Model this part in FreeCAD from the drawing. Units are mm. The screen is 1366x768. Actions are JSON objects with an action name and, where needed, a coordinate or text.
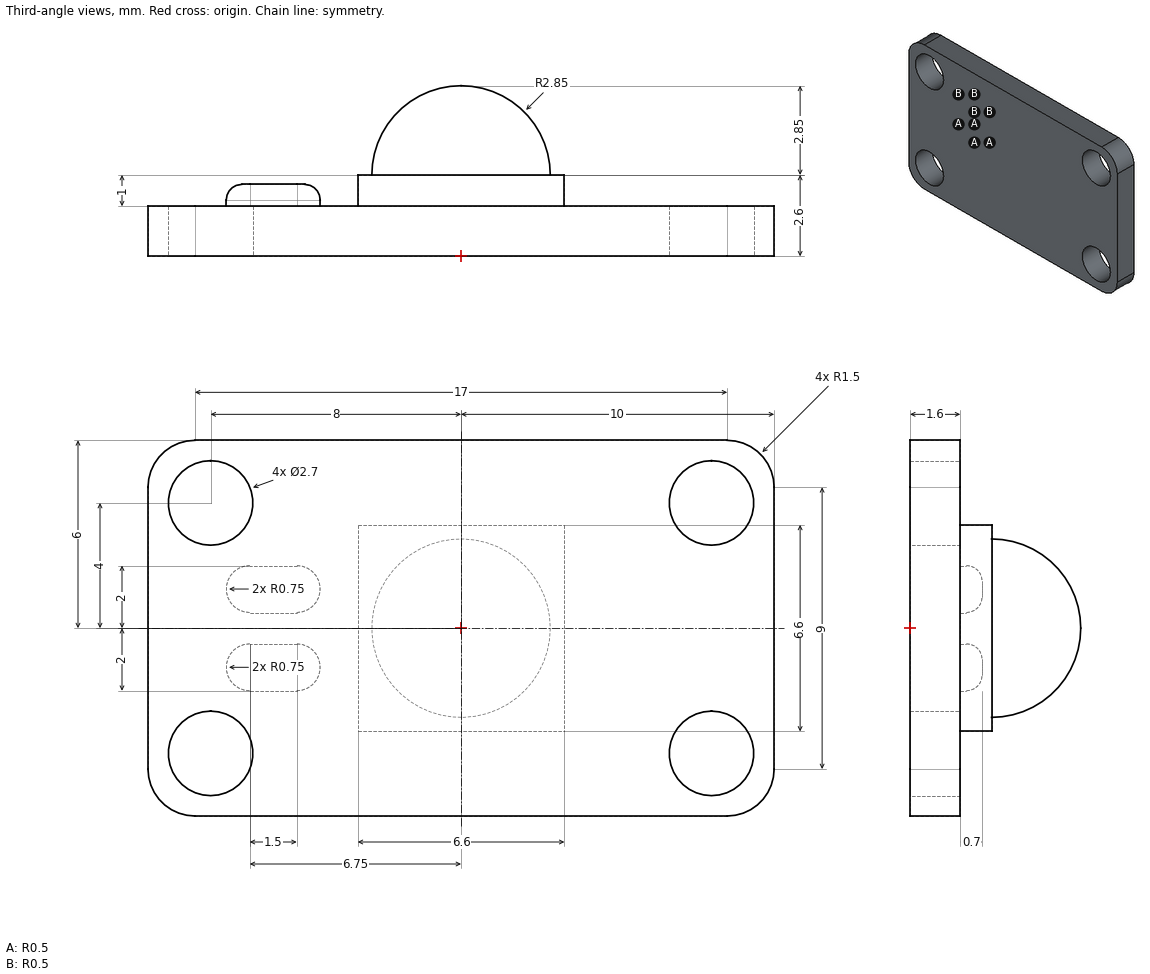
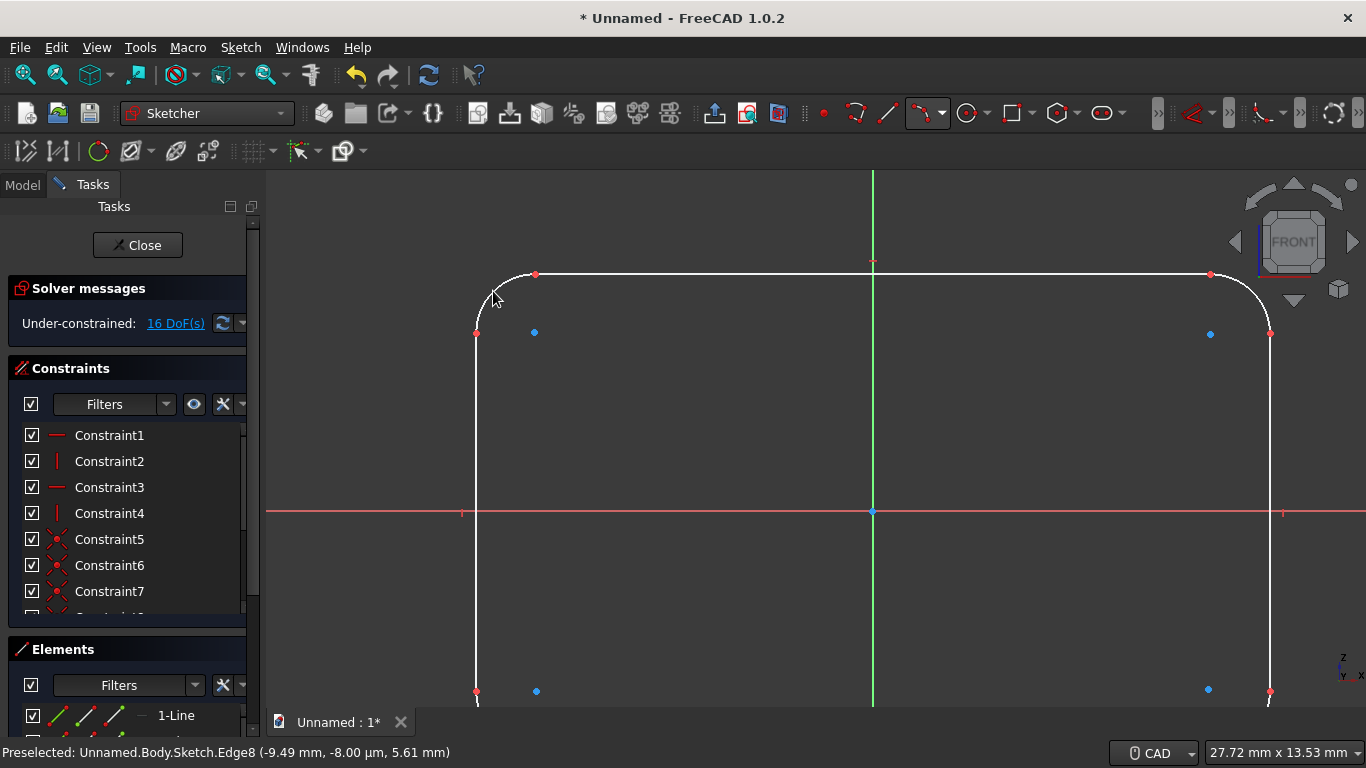
{"action": "left_click", "coordinate": [738, 274]}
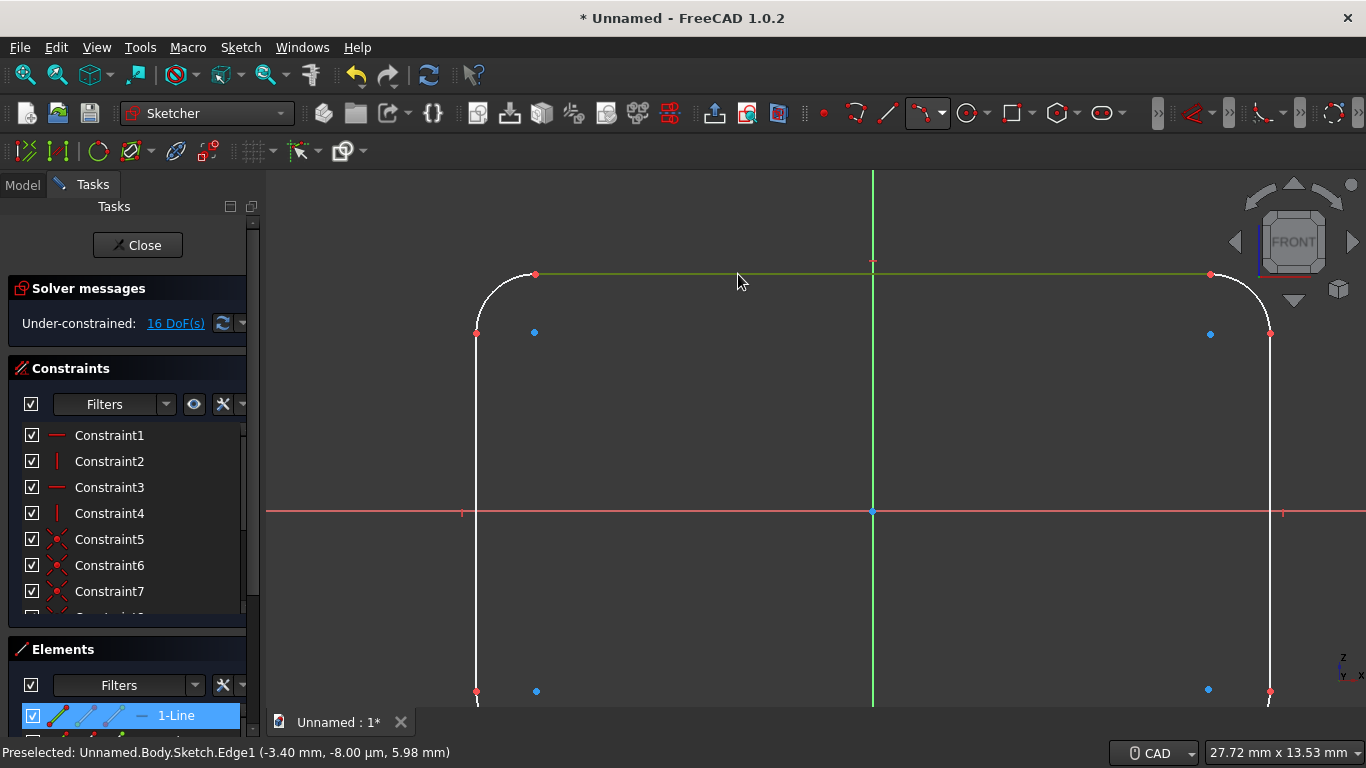
{"action": "scroll", "coordinate": [493, 290], "scroll_direction": "down", "scroll_amount": 2}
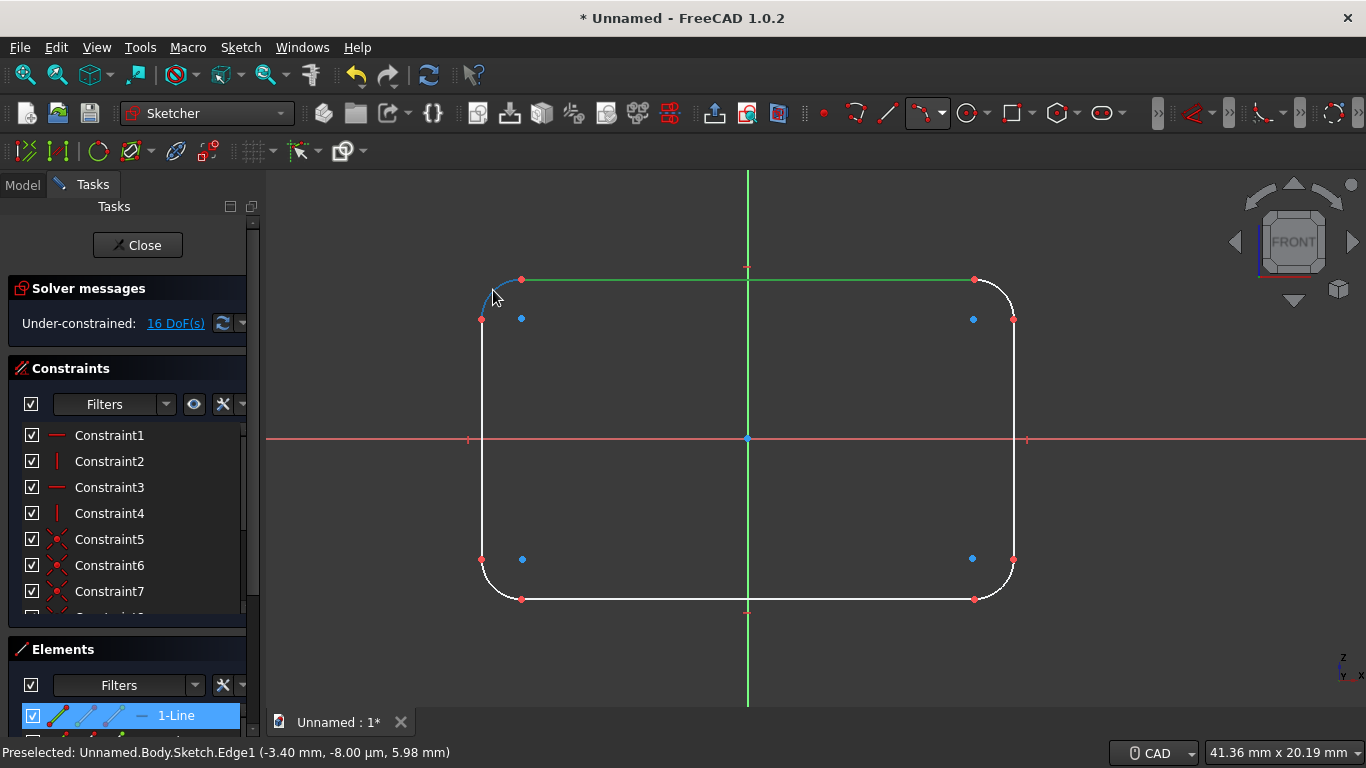
{"action": "left_click", "coordinate": [1010, 301]}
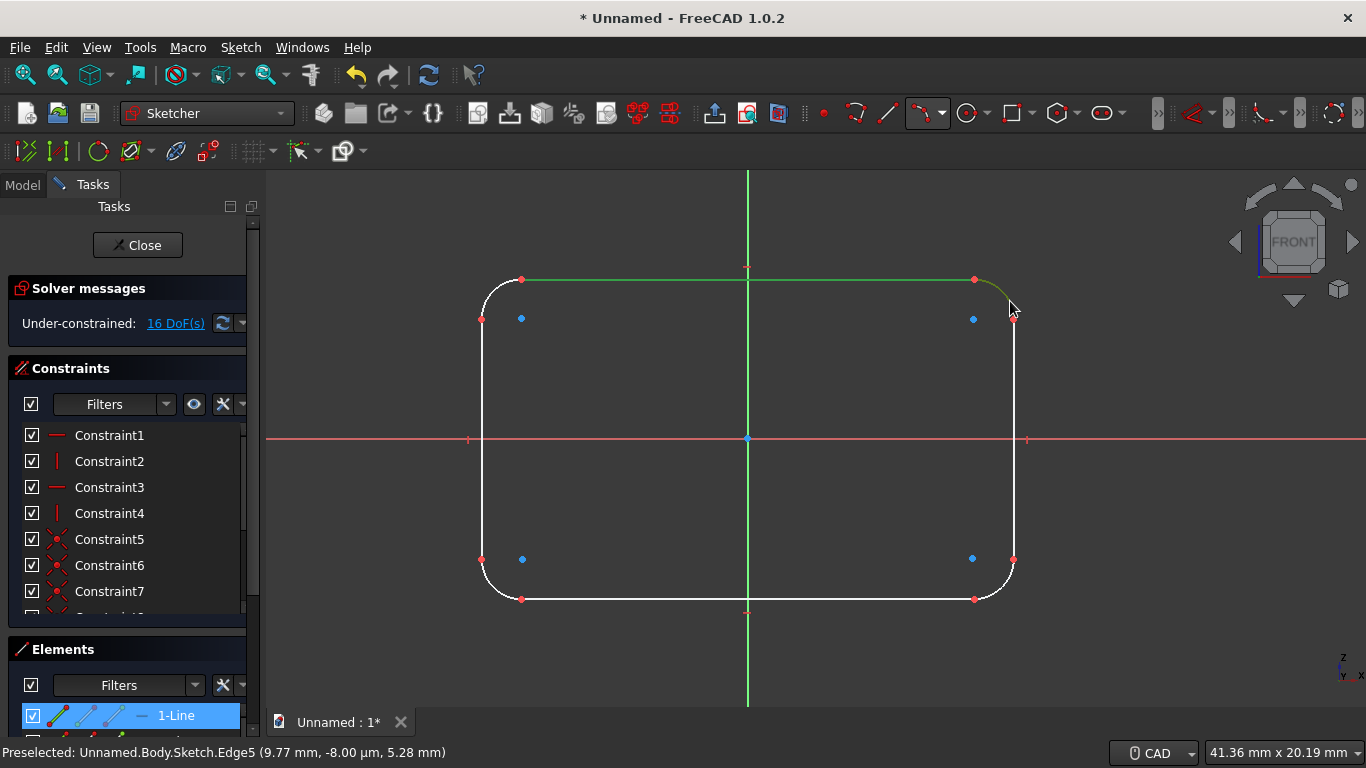
{"action": "key", "text": "t"}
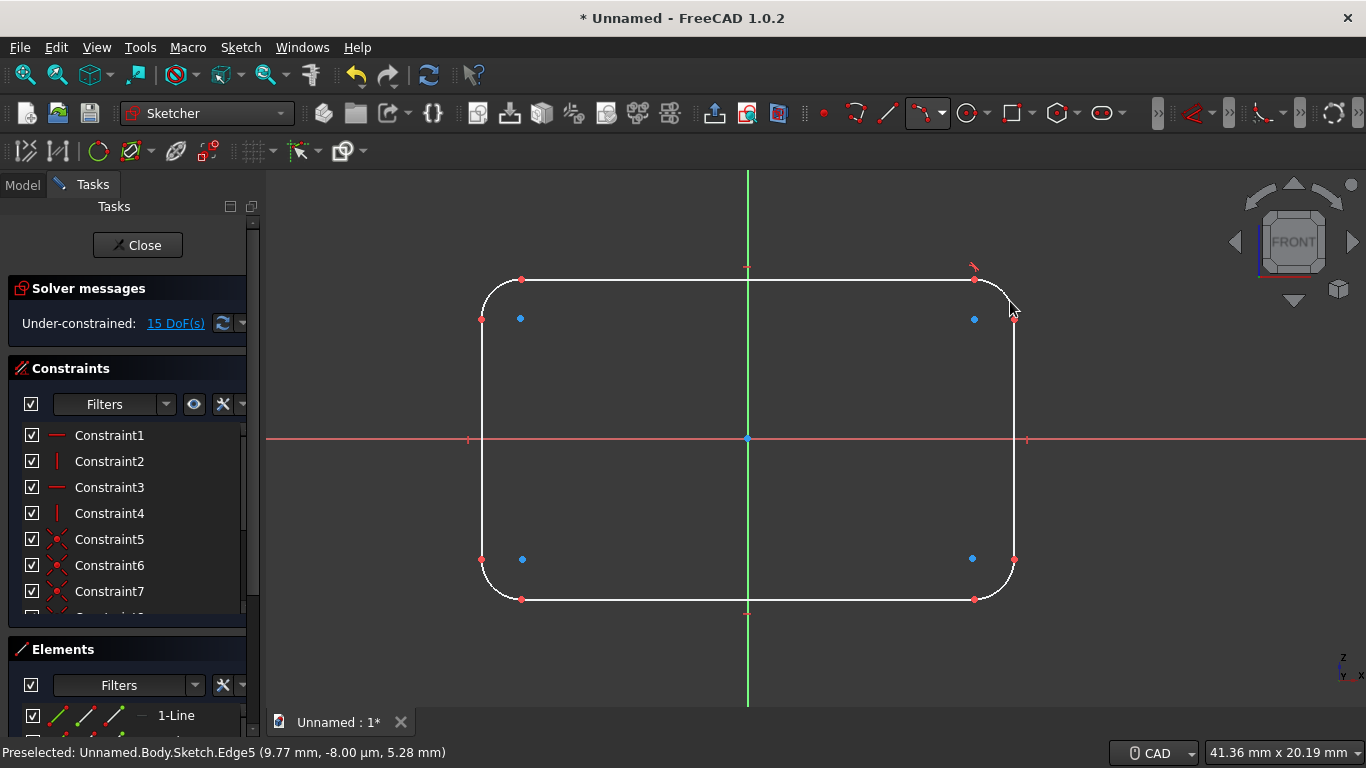
{"action": "left_click", "coordinate": [657, 280]}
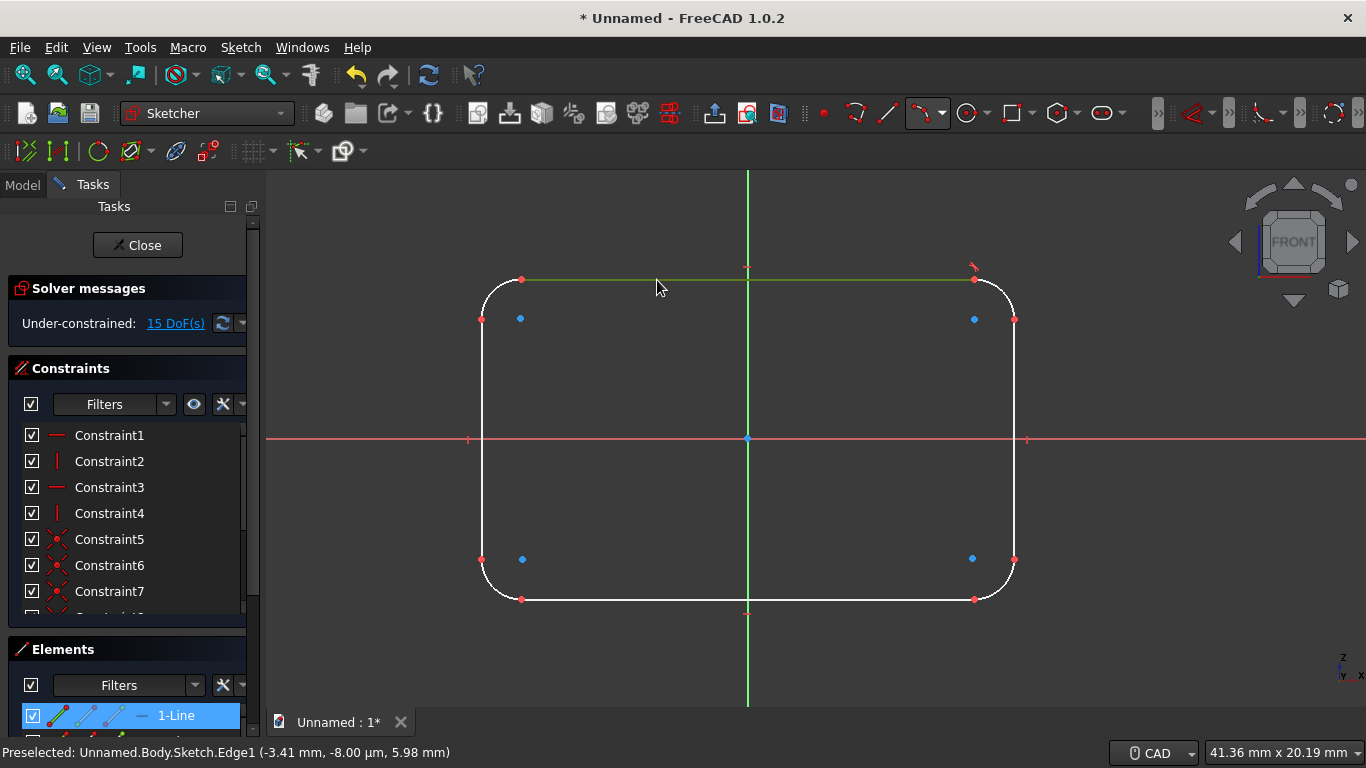
{"action": "left_click", "coordinate": [503, 284]}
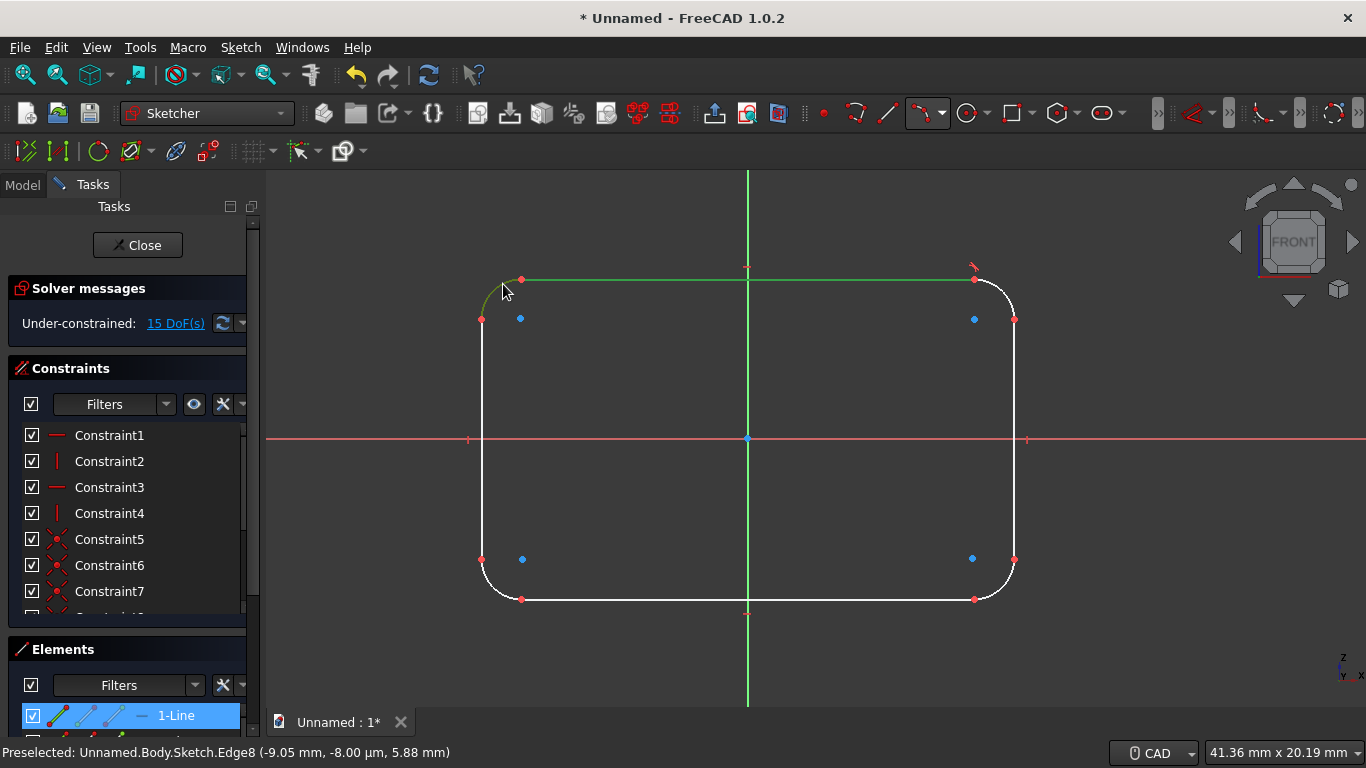
{"action": "key", "text": "t"}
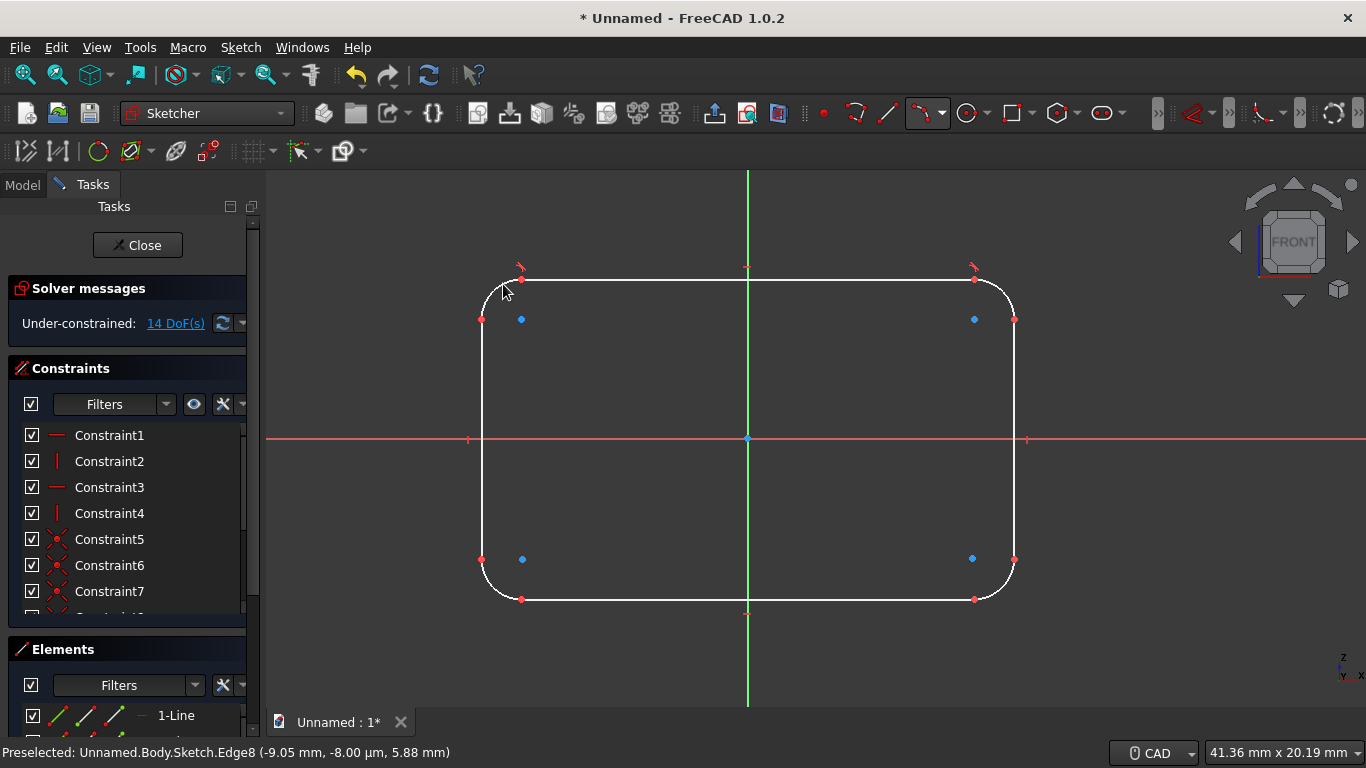
{"action": "left_click", "coordinate": [1014, 391]}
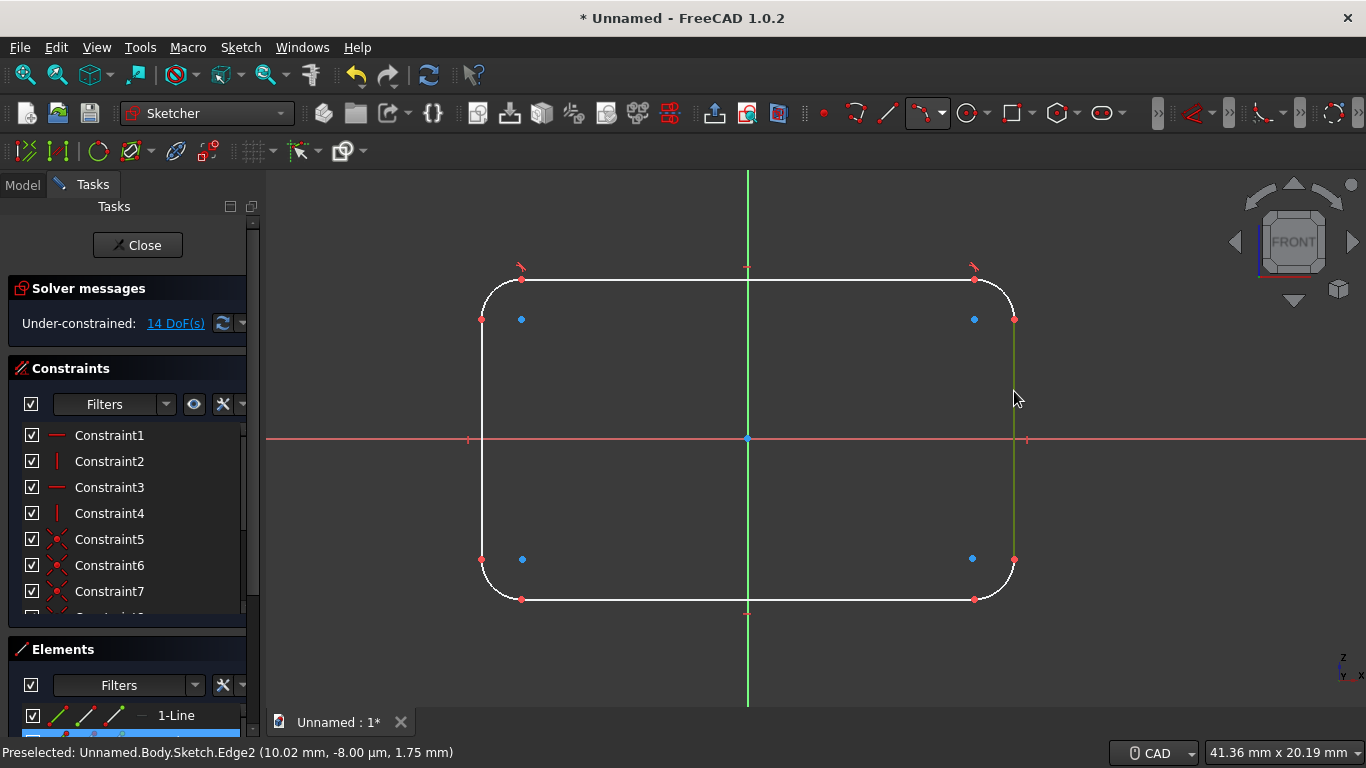
{"action": "left_click", "coordinate": [1010, 301]}